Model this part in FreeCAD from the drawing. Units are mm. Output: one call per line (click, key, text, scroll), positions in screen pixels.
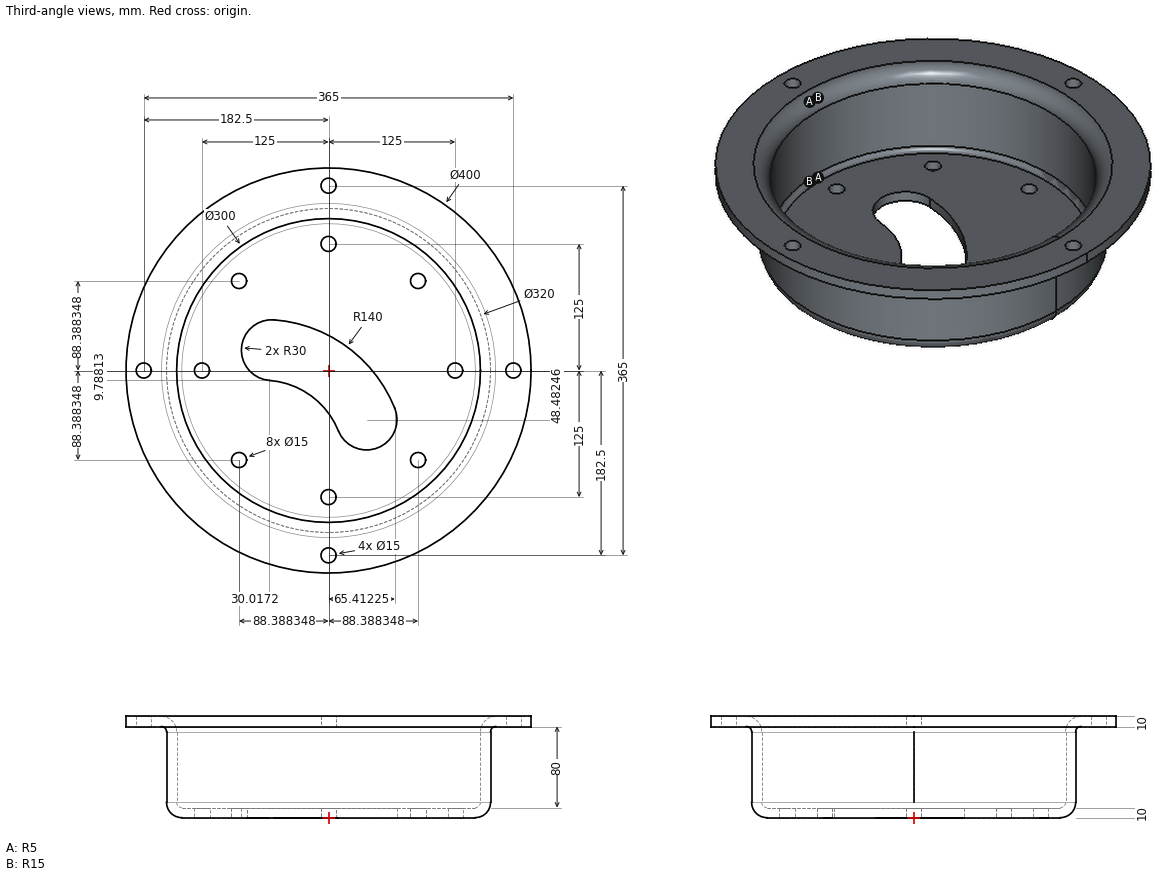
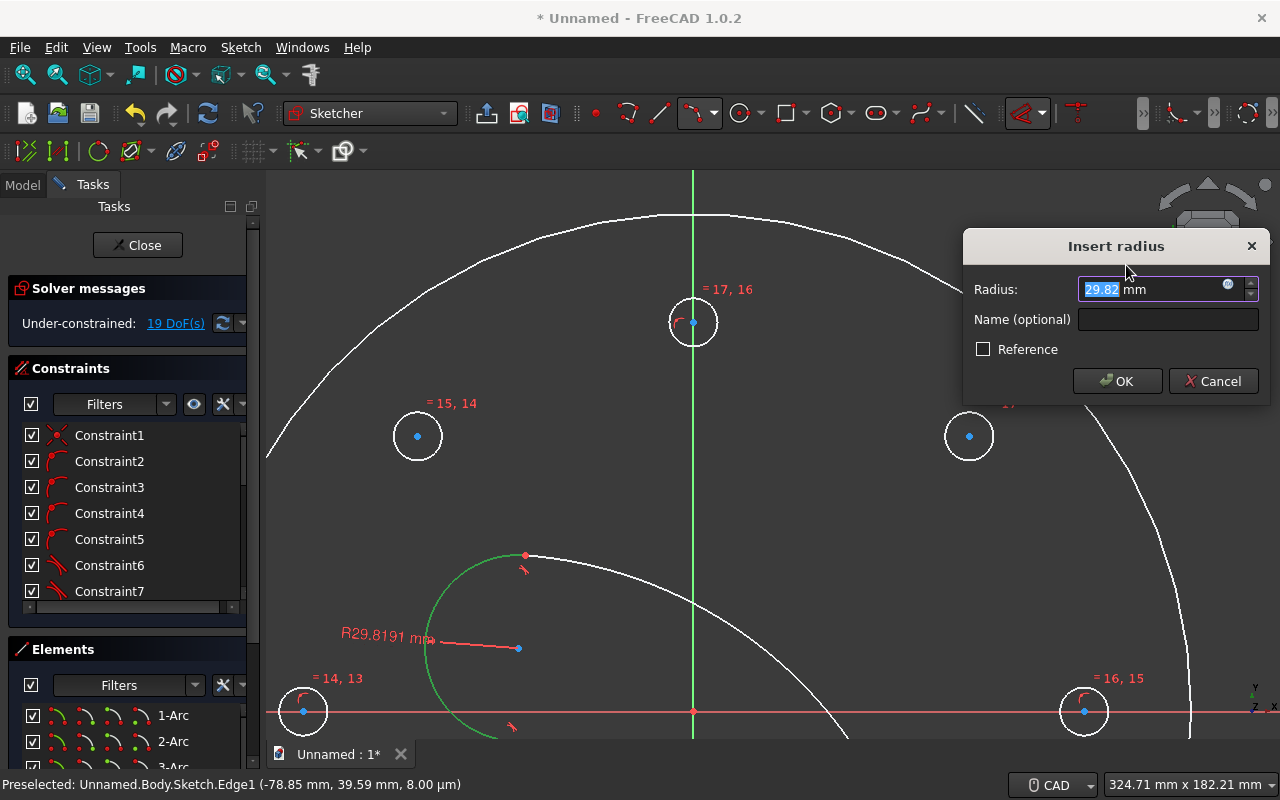
text(30)
key(Return)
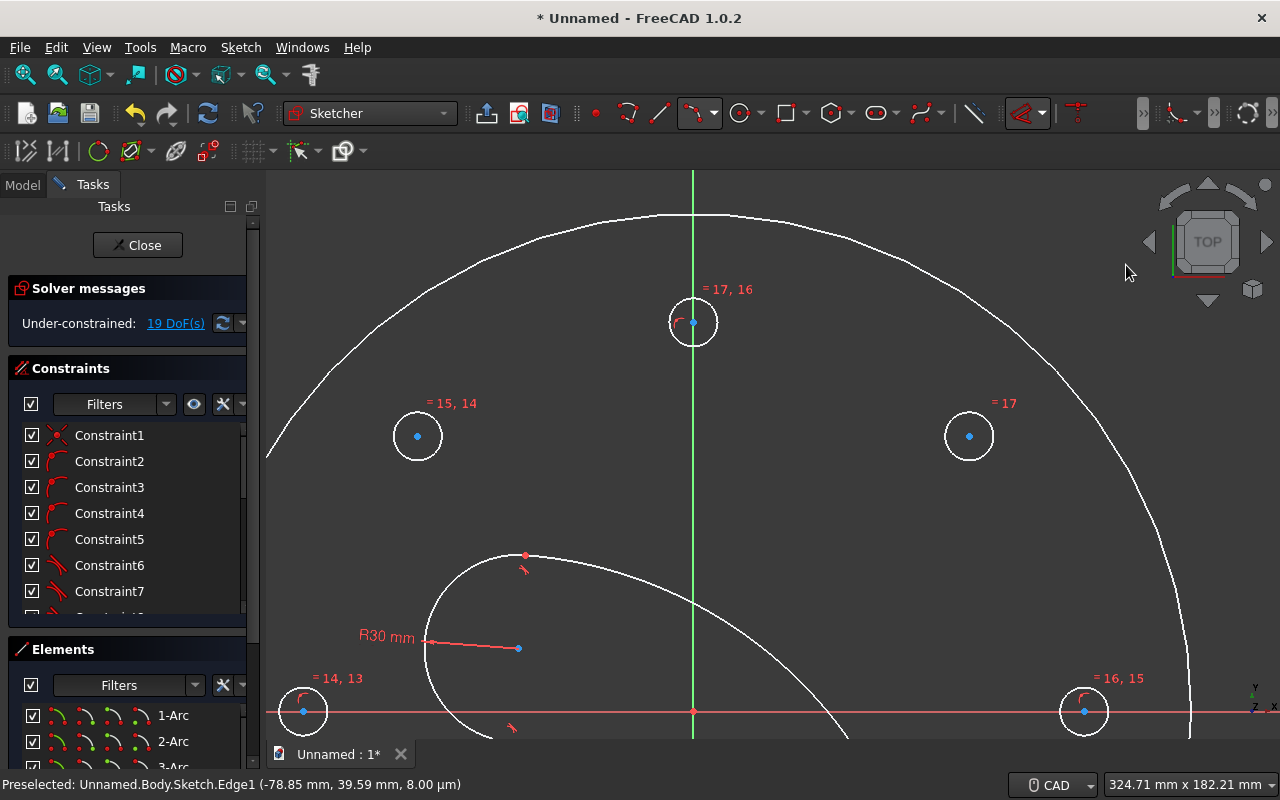
click(666, 590)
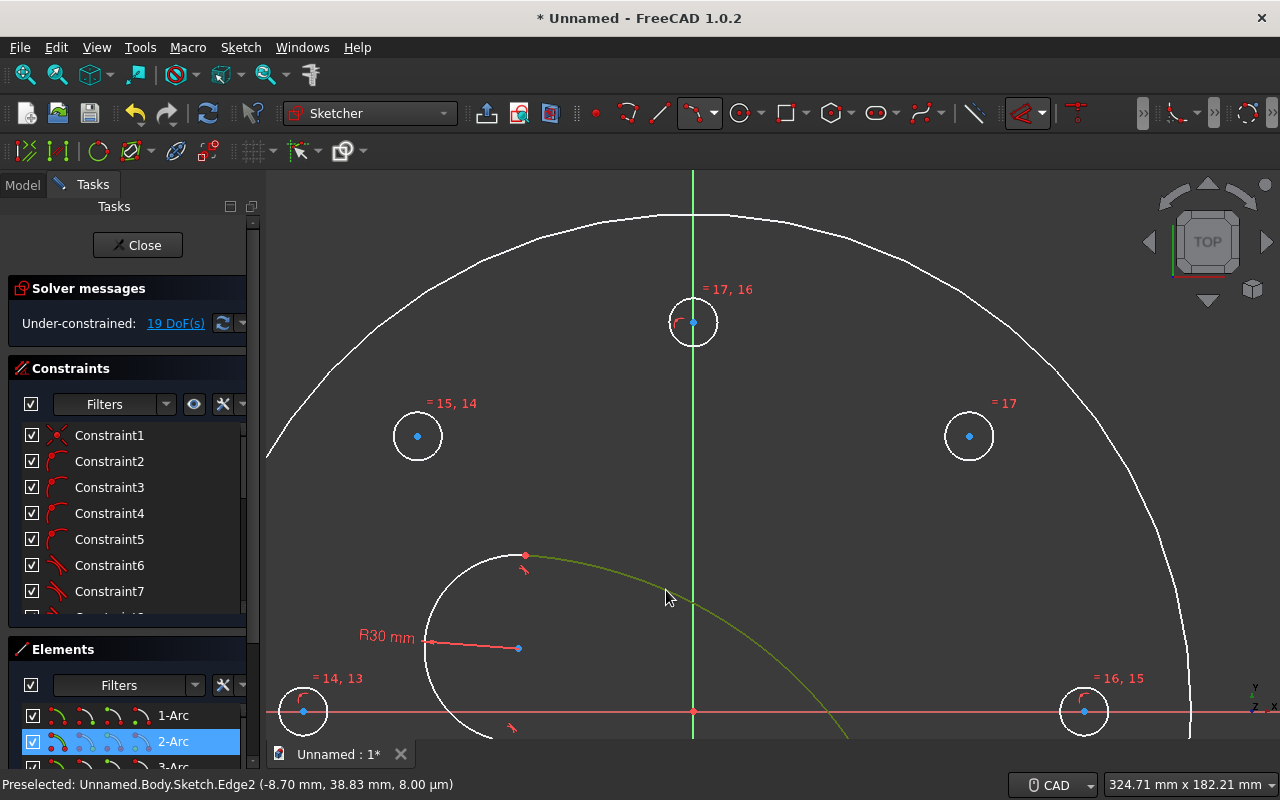
click(1044, 114)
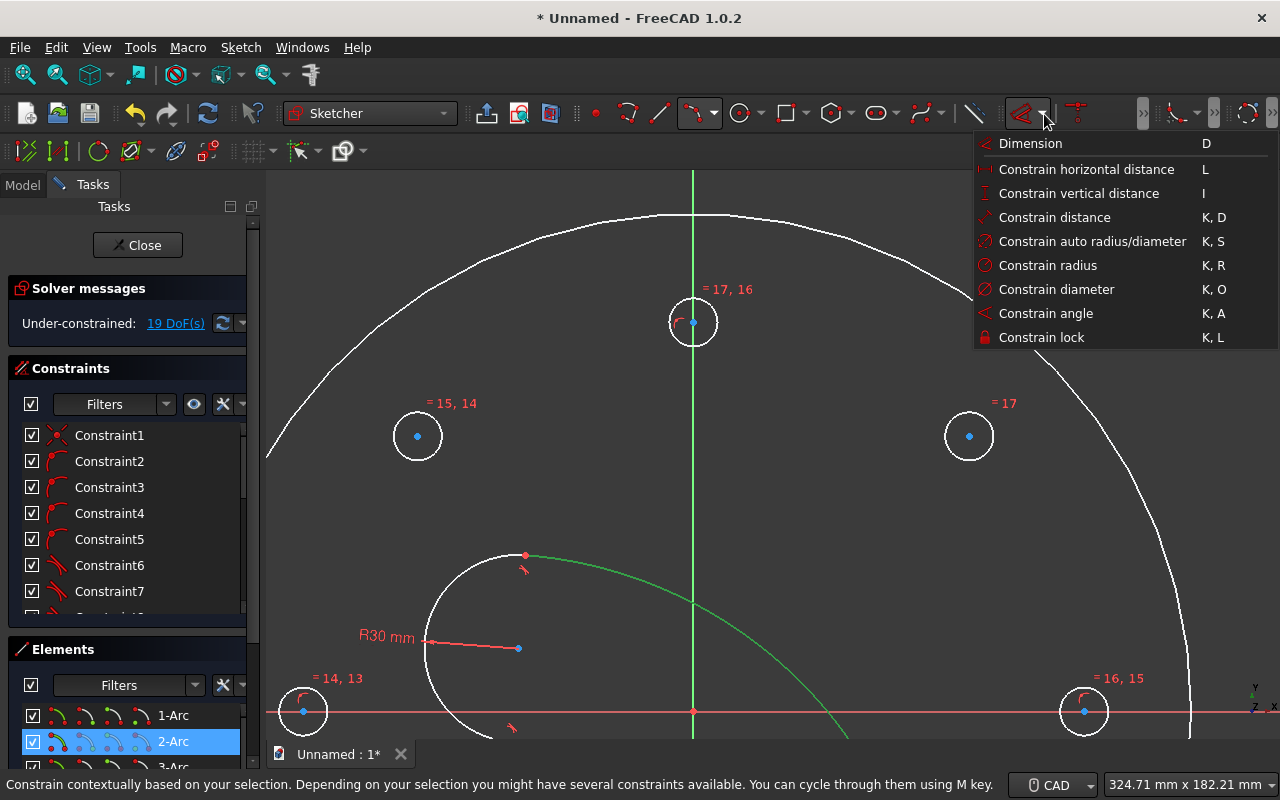
click(1126, 265)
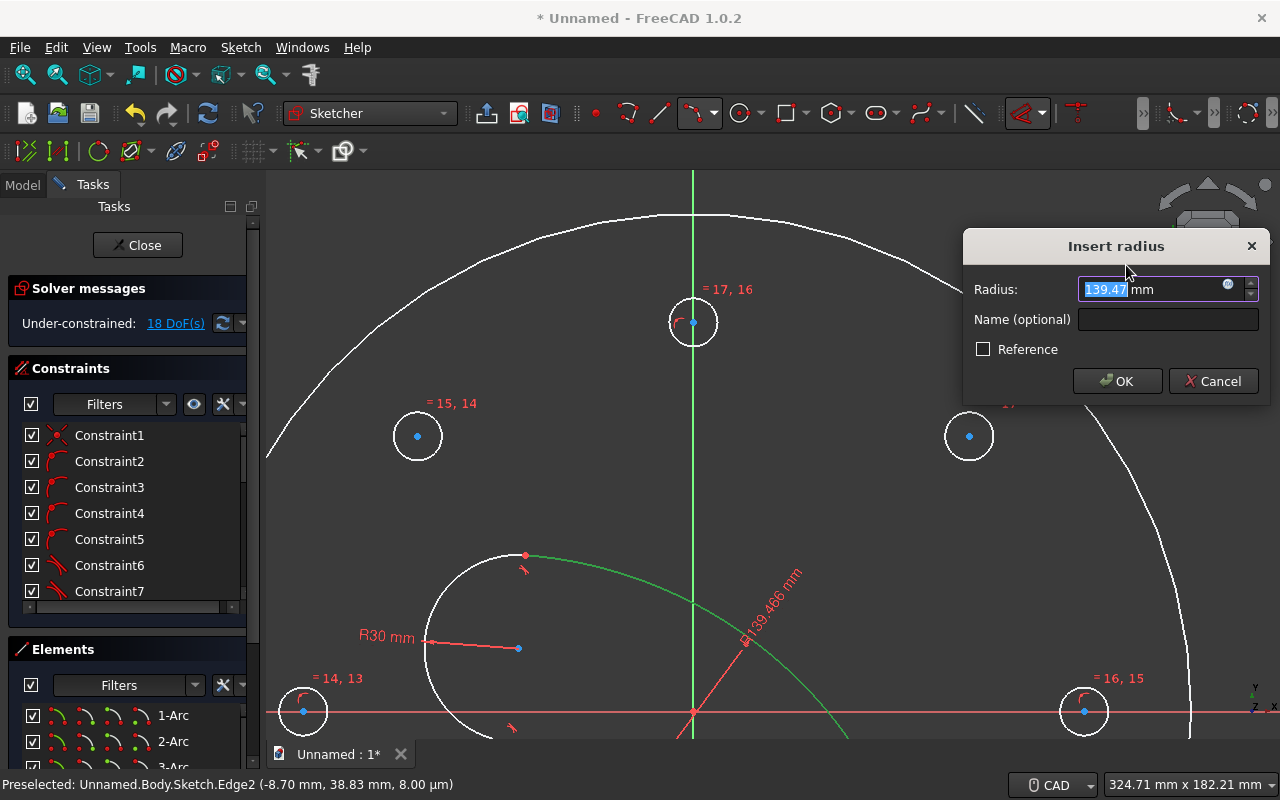
text(140)
key(Return)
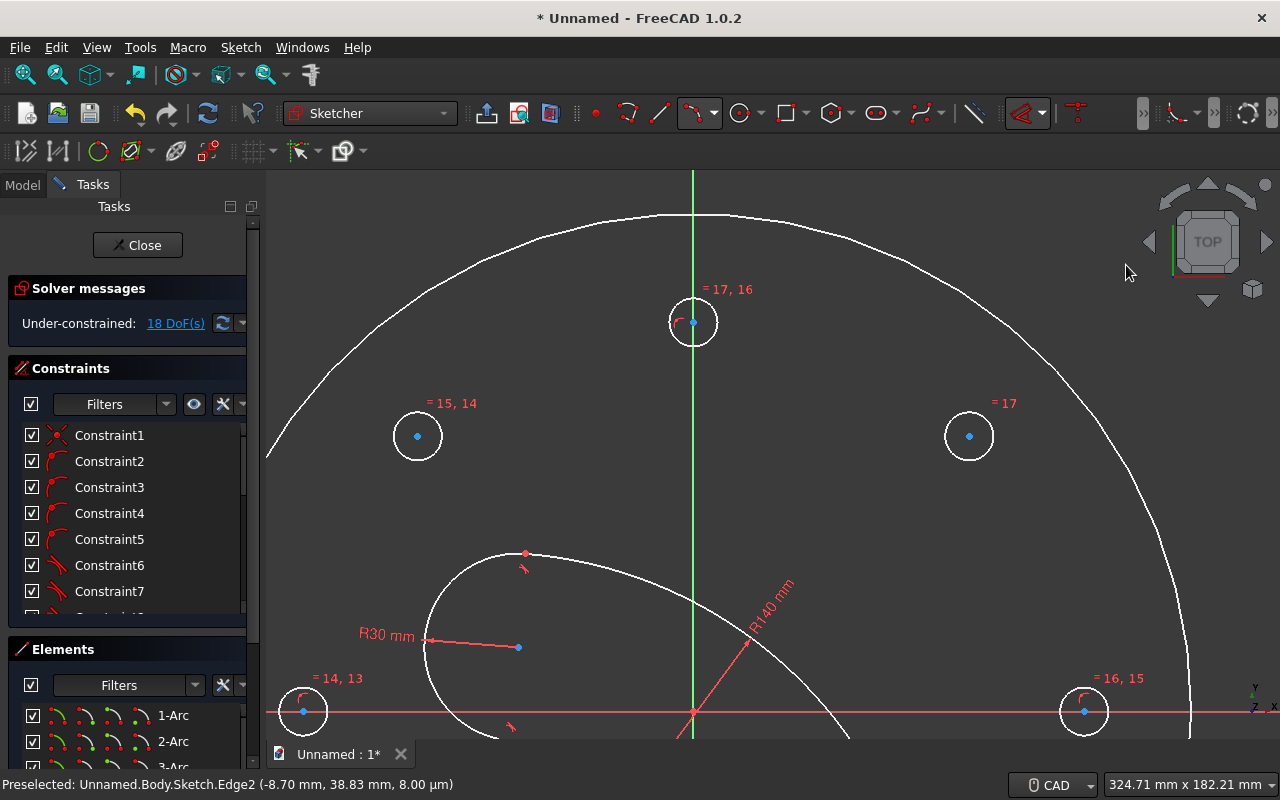
click(1044, 359)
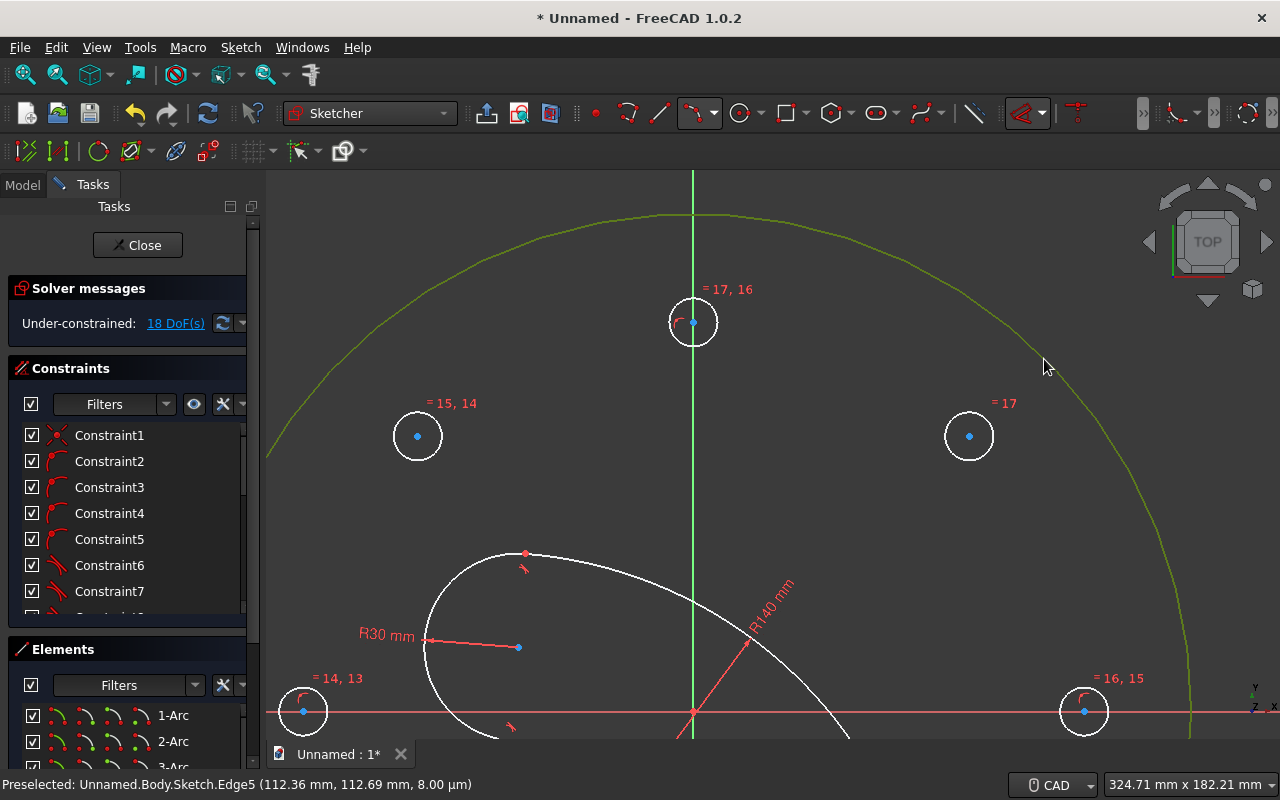
key(k)
key(o)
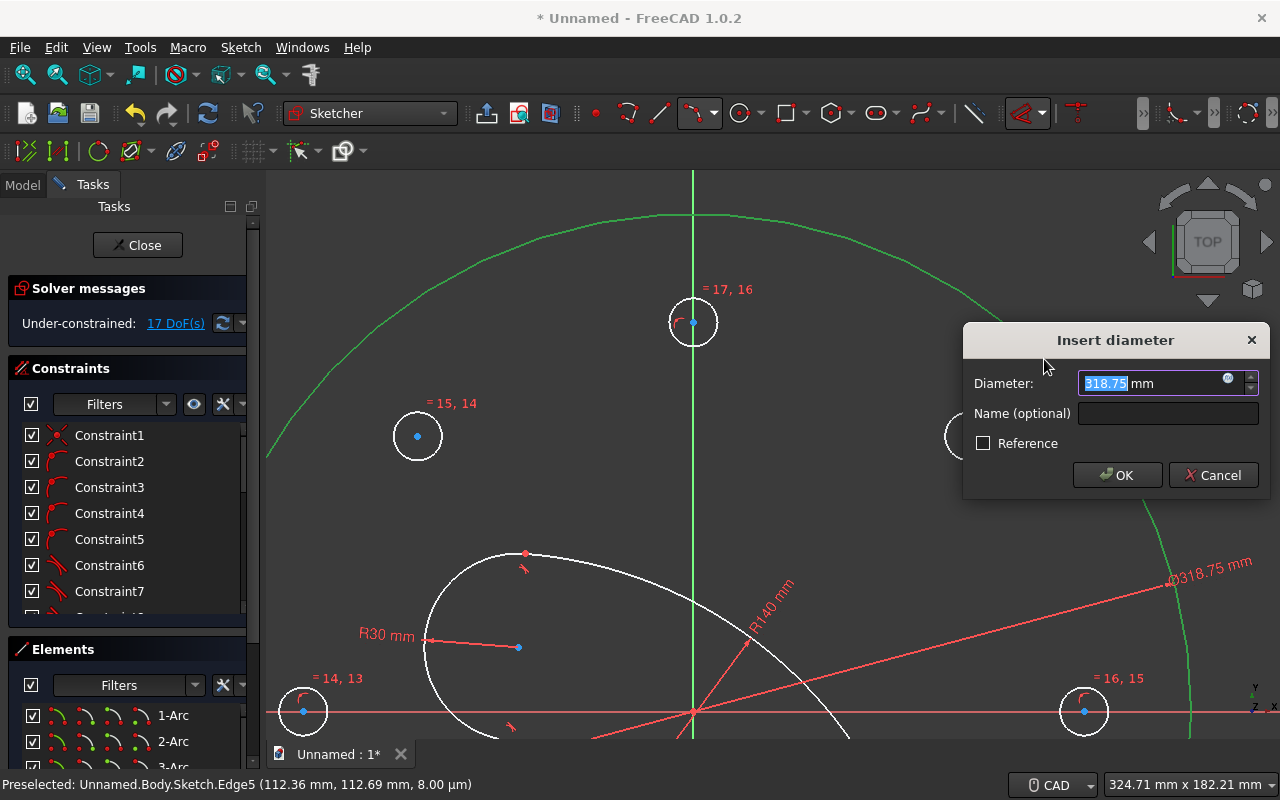
text(320)
key(Return)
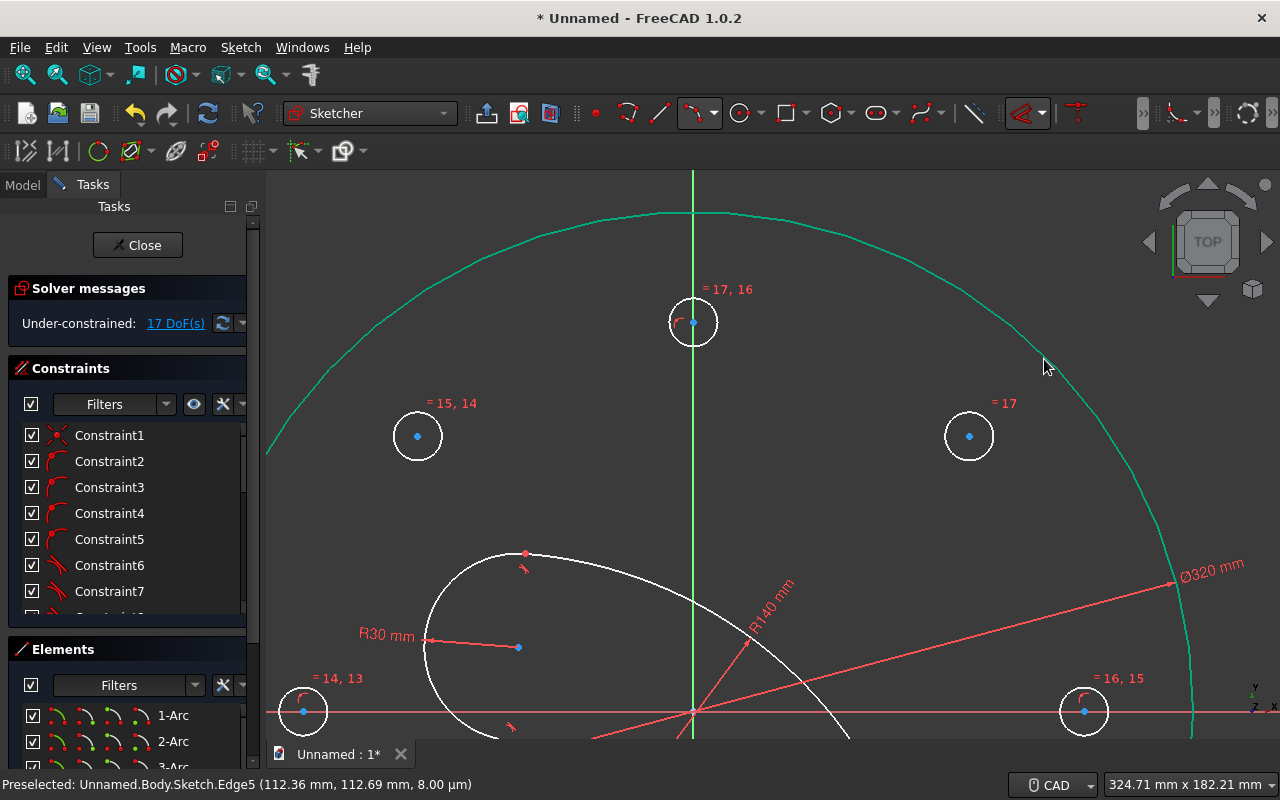
scroll(711, 305, down, 5)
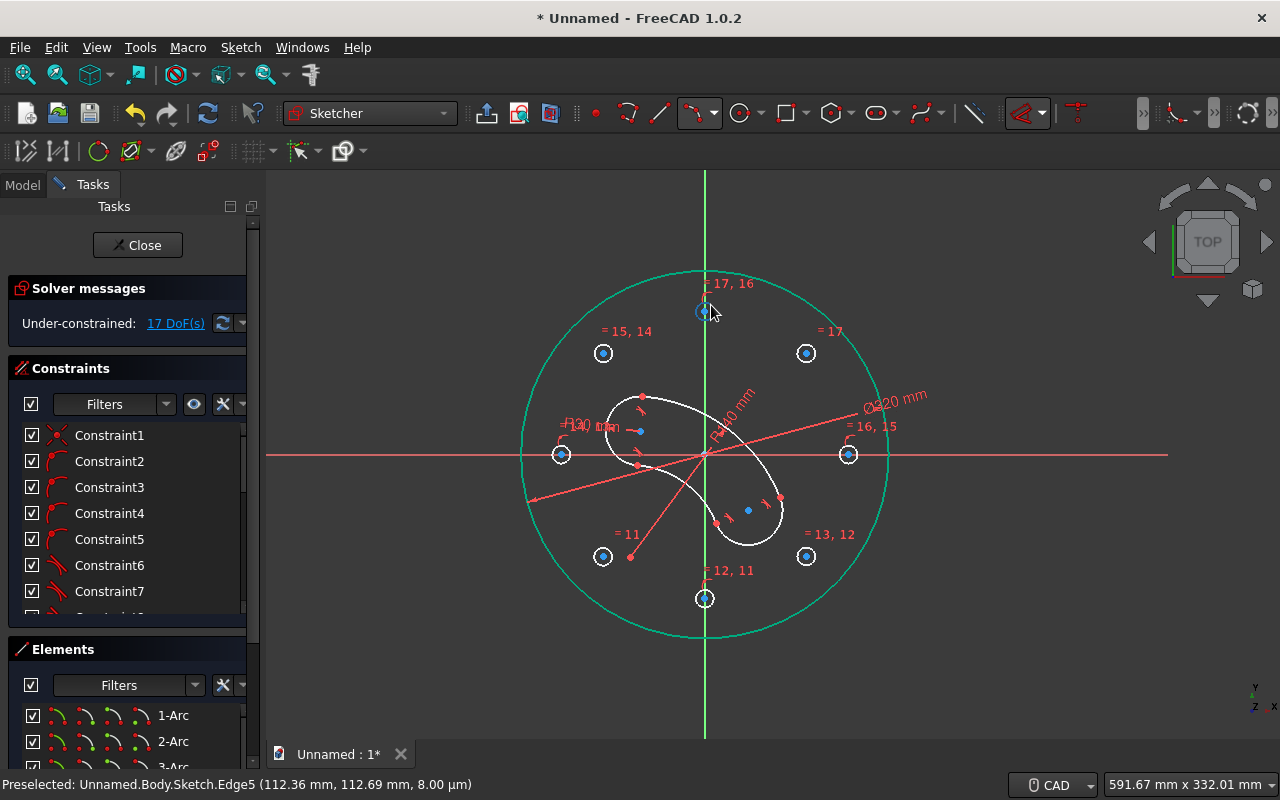
scroll(609, 551, up, 5)